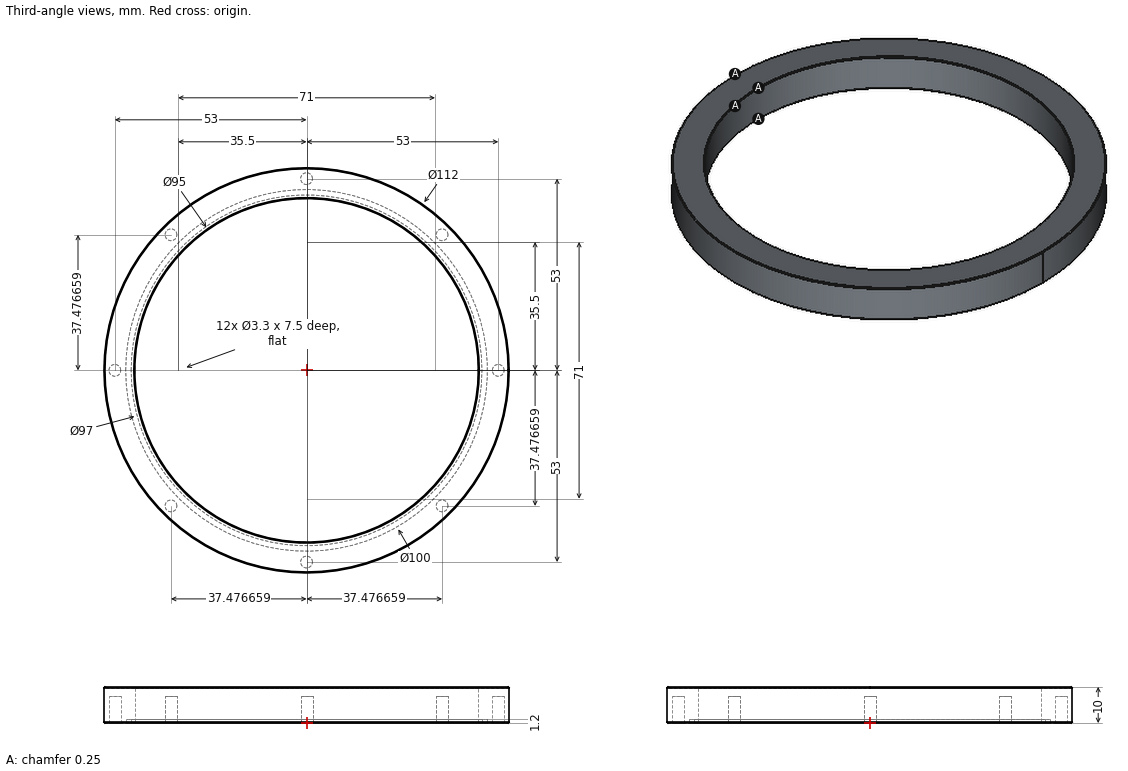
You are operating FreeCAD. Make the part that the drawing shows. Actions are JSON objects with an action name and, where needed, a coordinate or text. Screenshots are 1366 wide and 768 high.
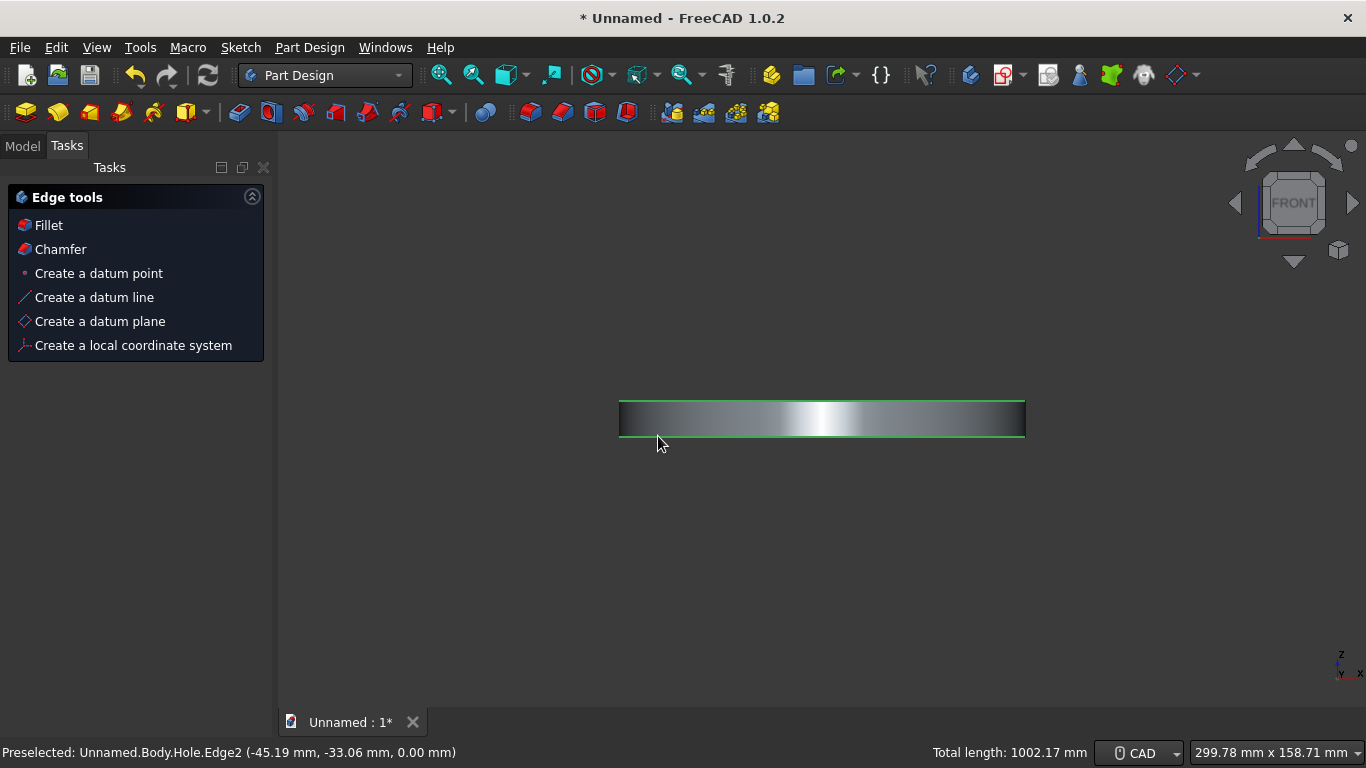
{"action": "key", "text": "3"}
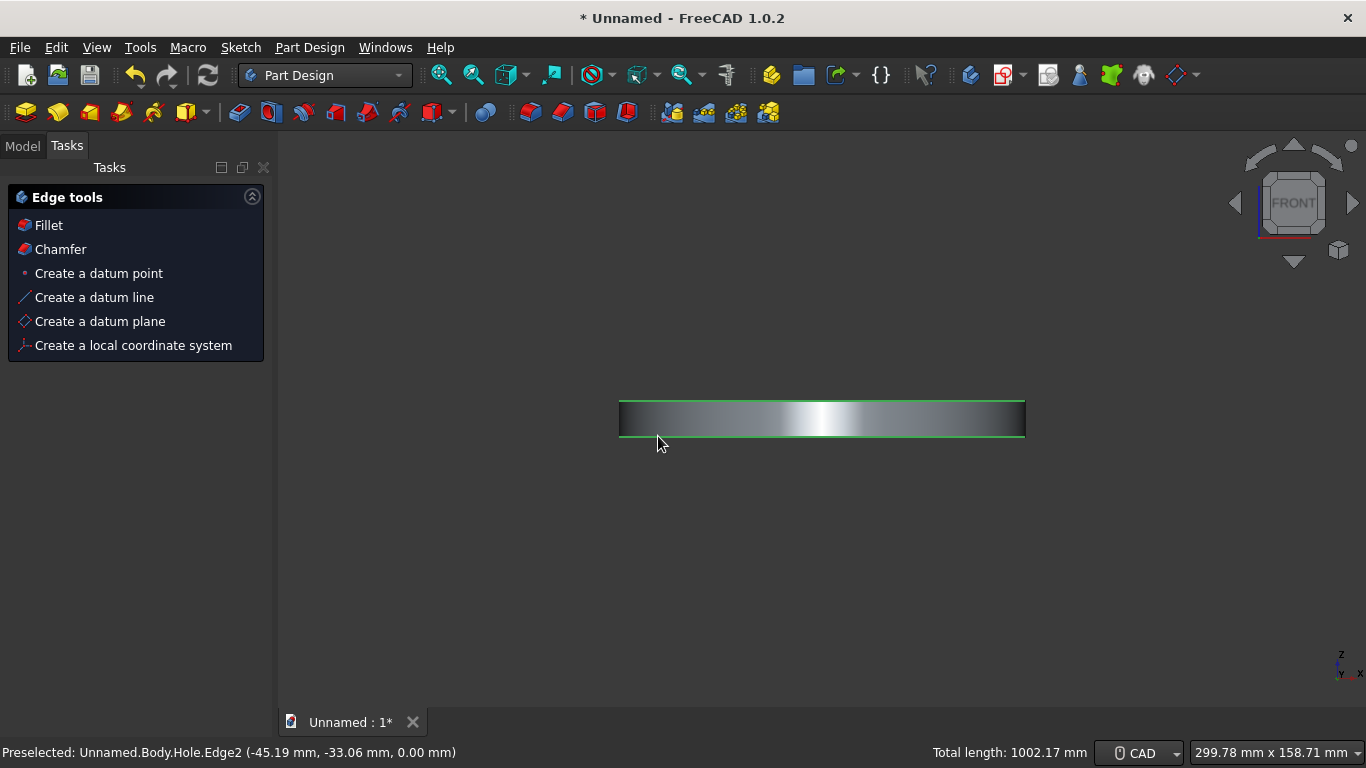
{"action": "left_click", "coordinate": [442, 76]}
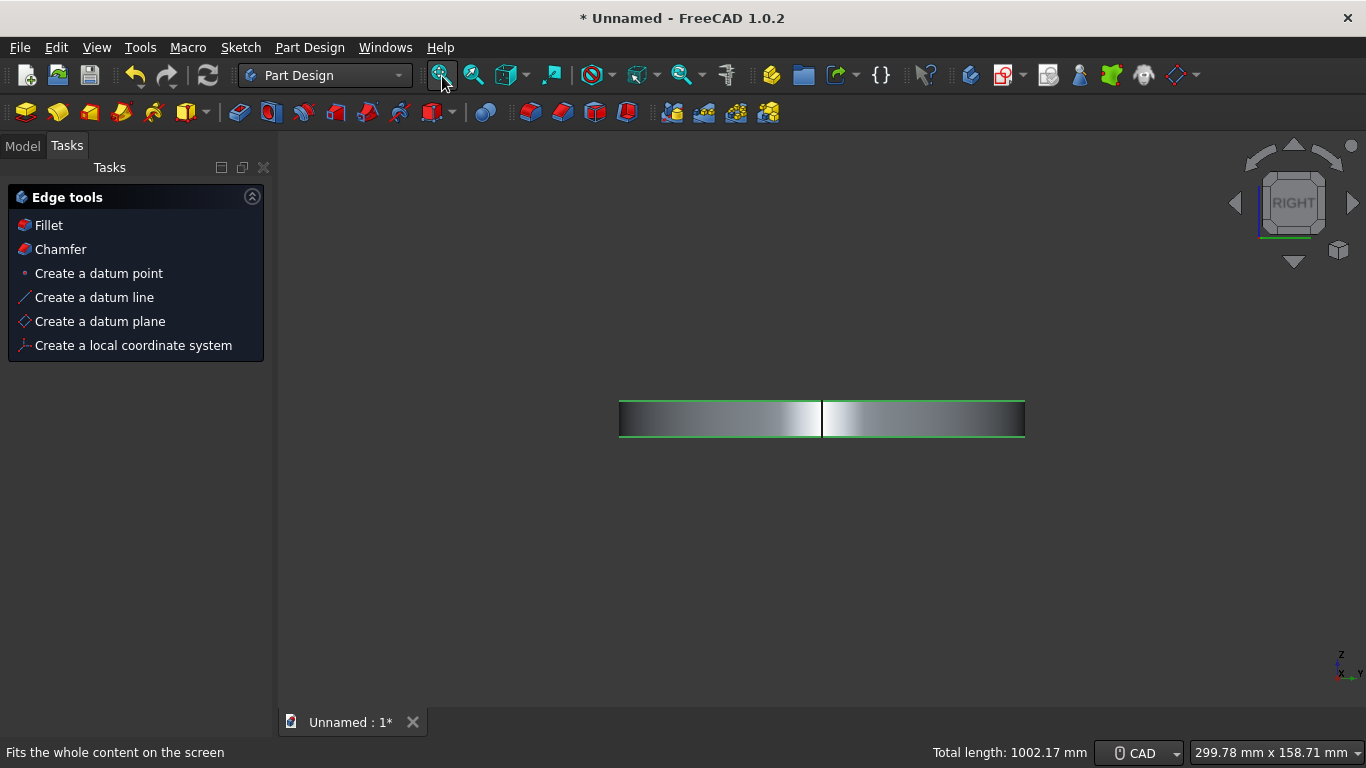
{"action": "key", "text": "5"}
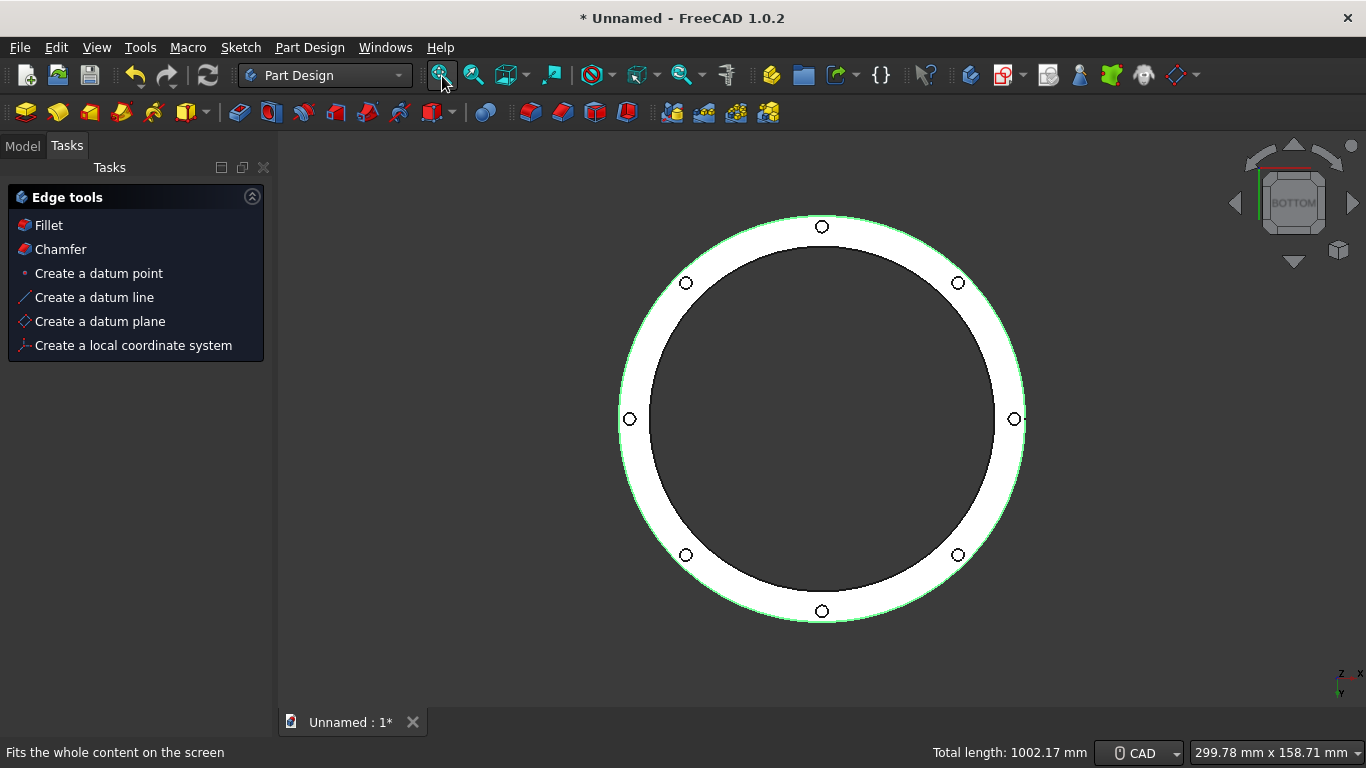
{"action": "left_click", "coordinate": [650, 418], "text": "ctrl"}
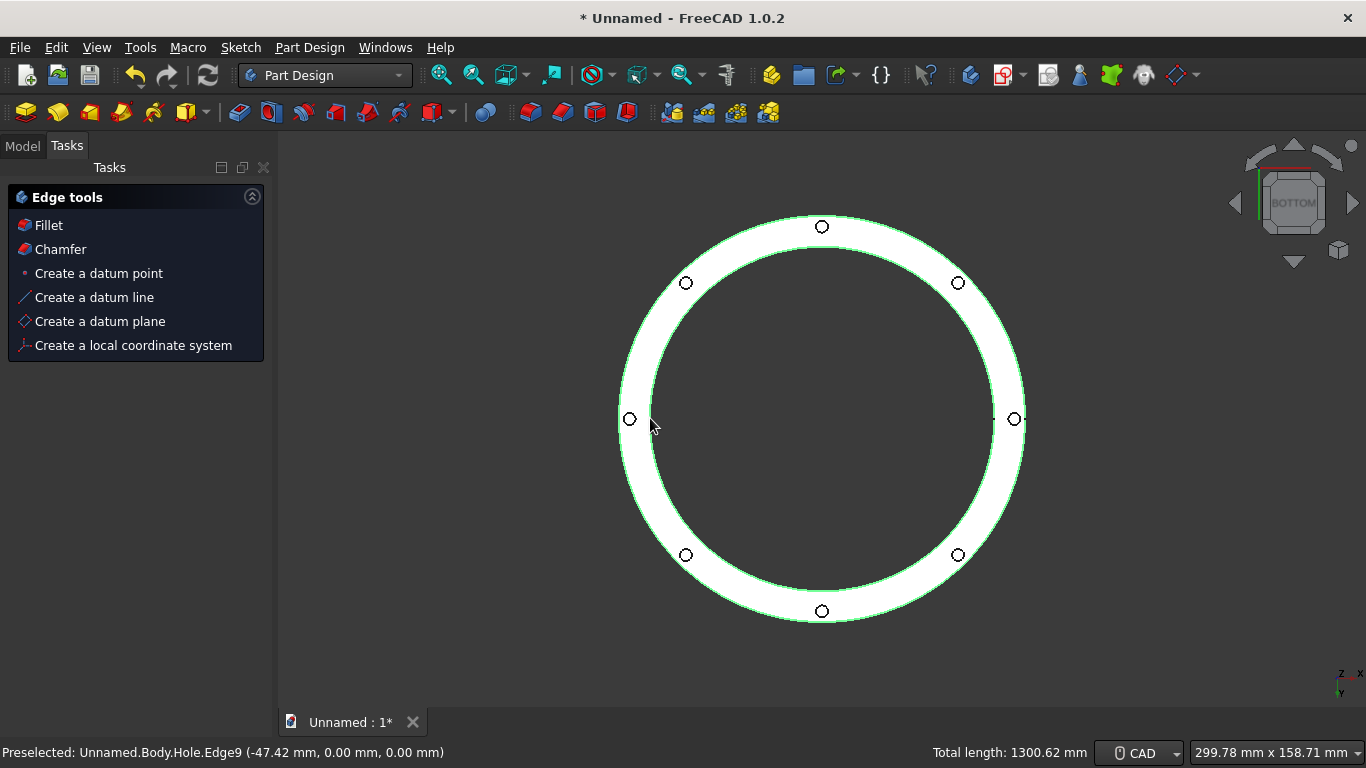
{"action": "left_click", "coordinate": [564, 112]}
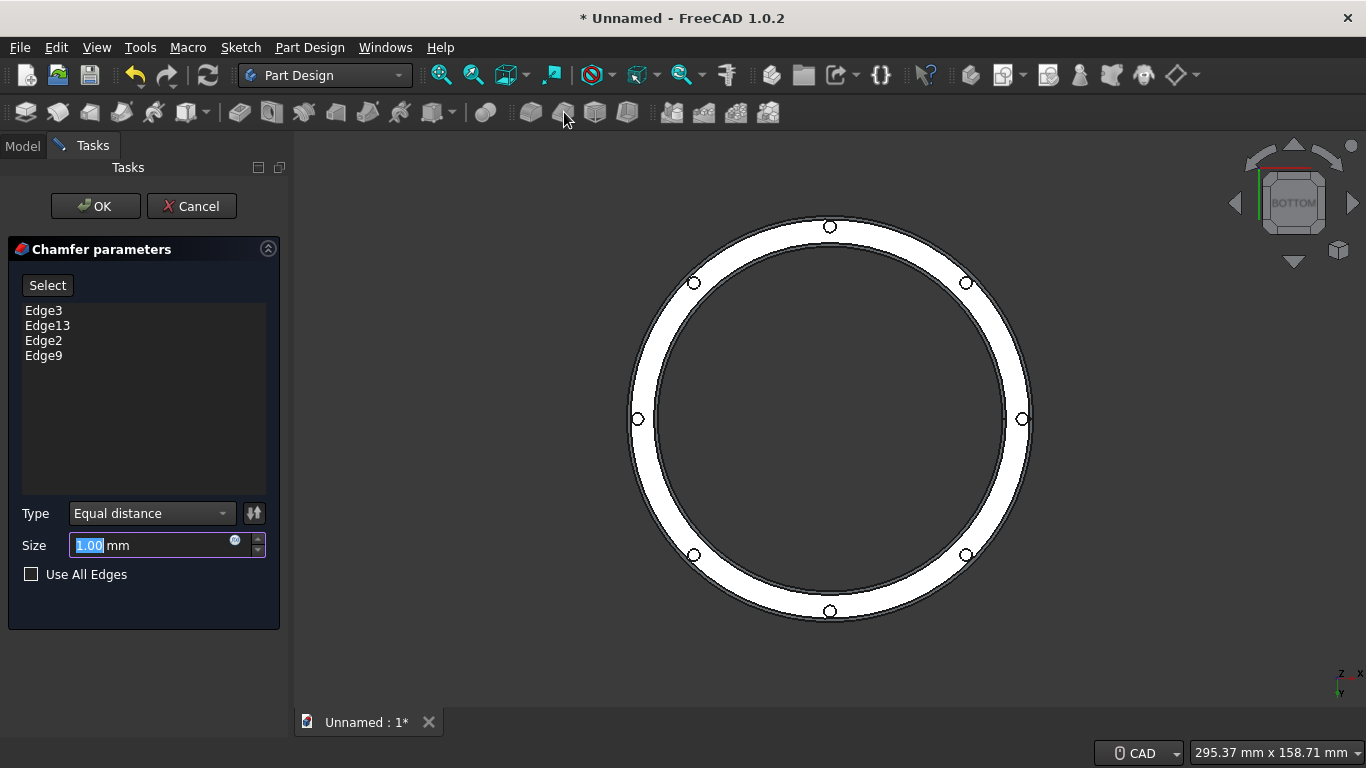
{"action": "type", "text": "0.25"}
{"action": "key", "text": "Tab"}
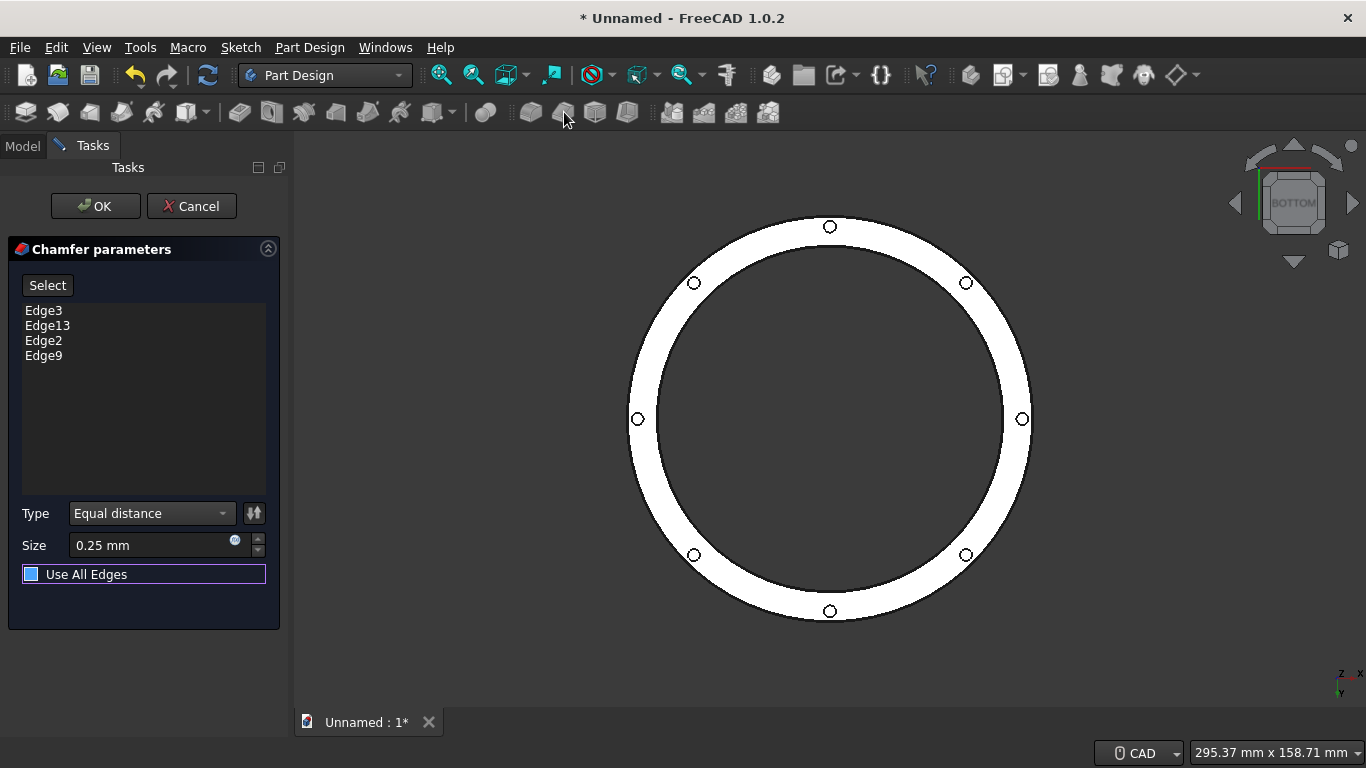
{"action": "left_click", "coordinate": [96, 206]}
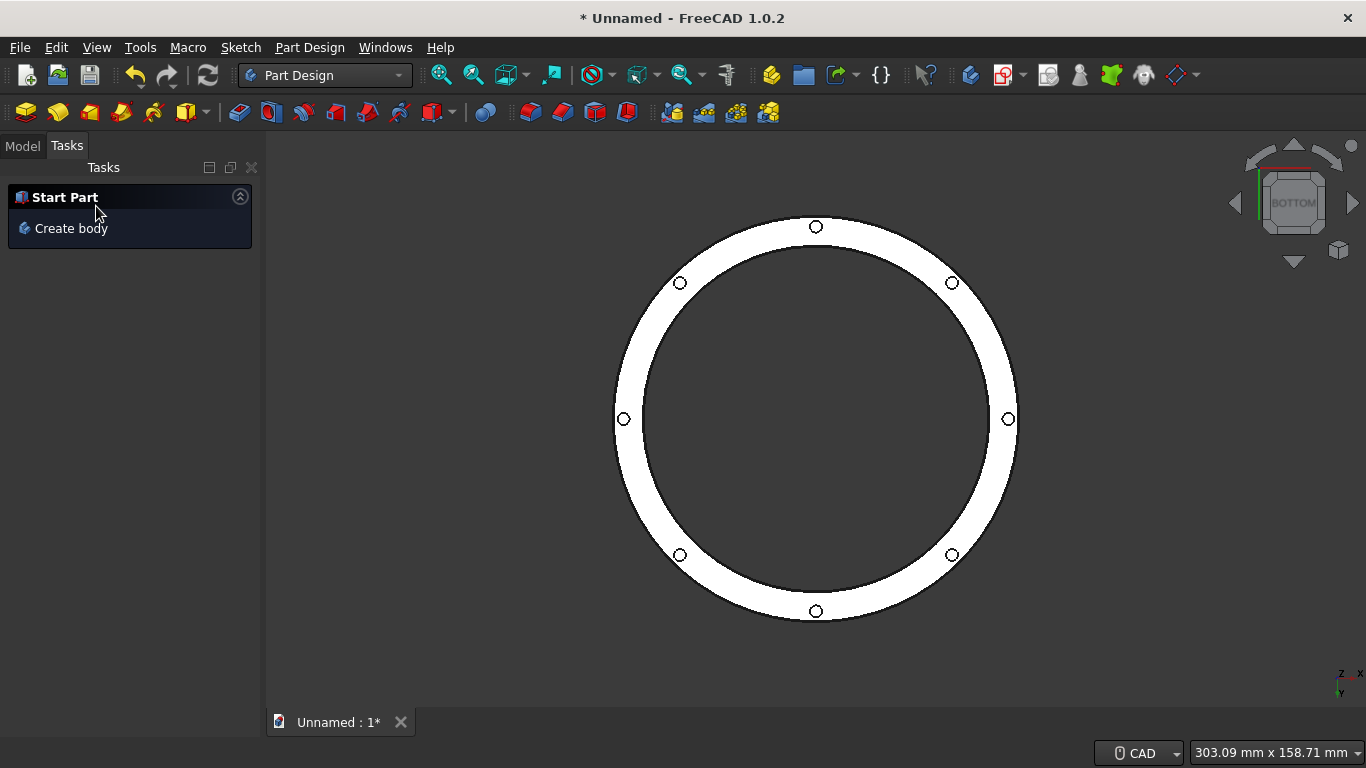
{"action": "left_click", "coordinate": [874, 591]}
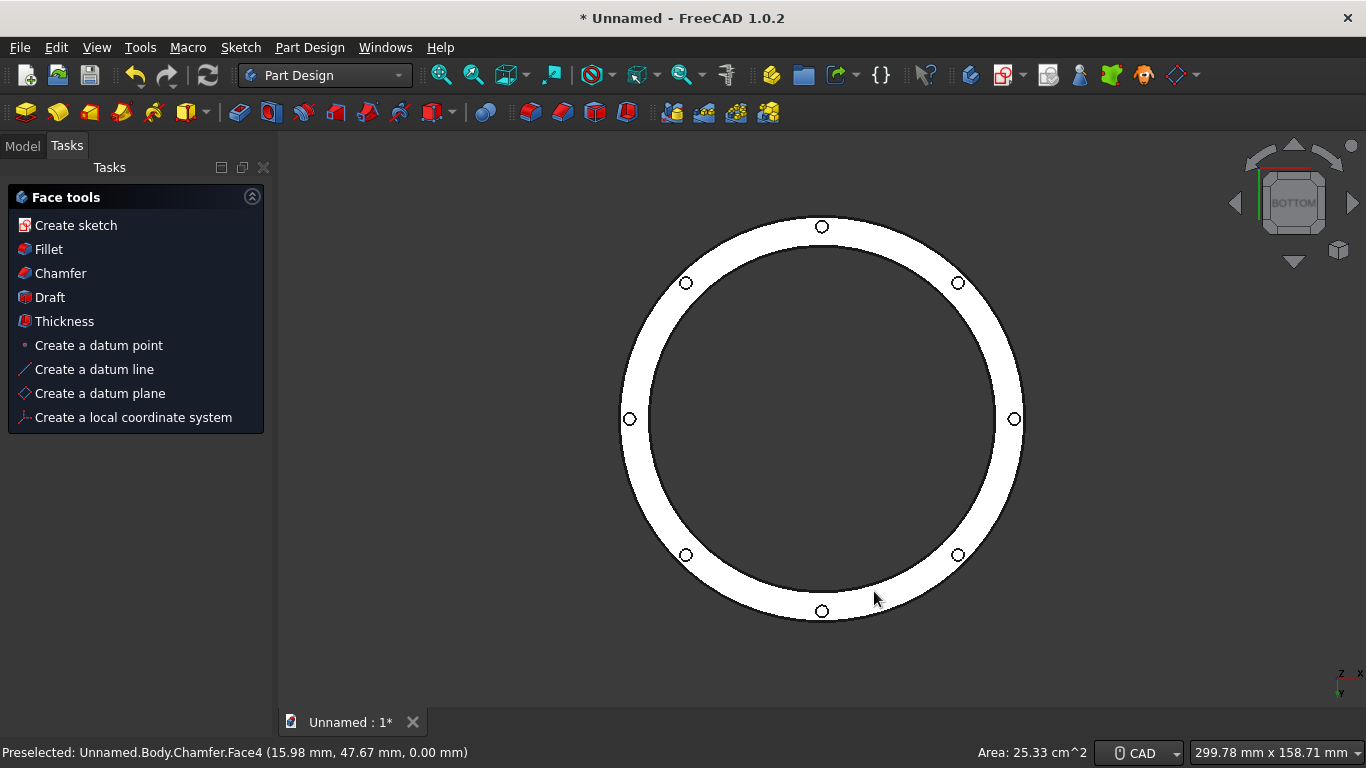
{"action": "left_click", "coordinate": [1004, 76]}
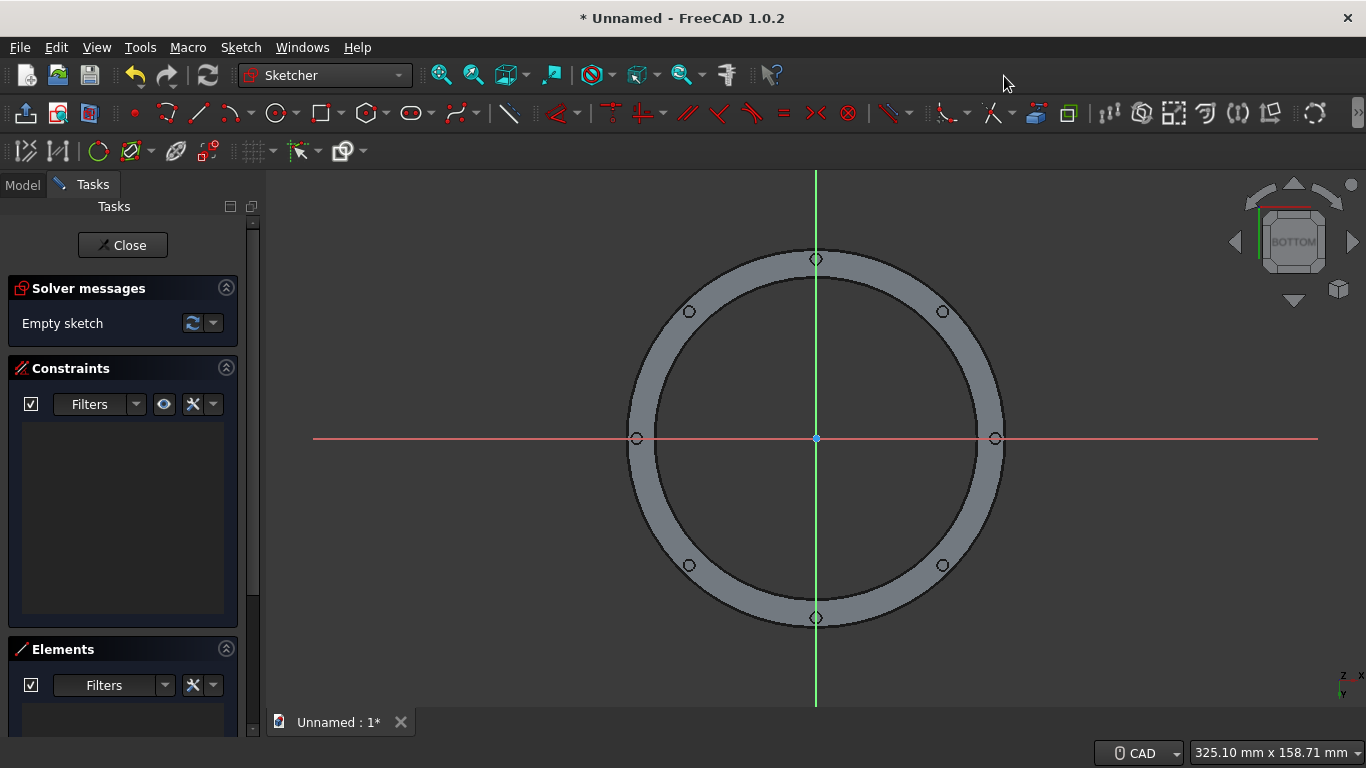
{"action": "left_click", "coordinate": [276, 114]}